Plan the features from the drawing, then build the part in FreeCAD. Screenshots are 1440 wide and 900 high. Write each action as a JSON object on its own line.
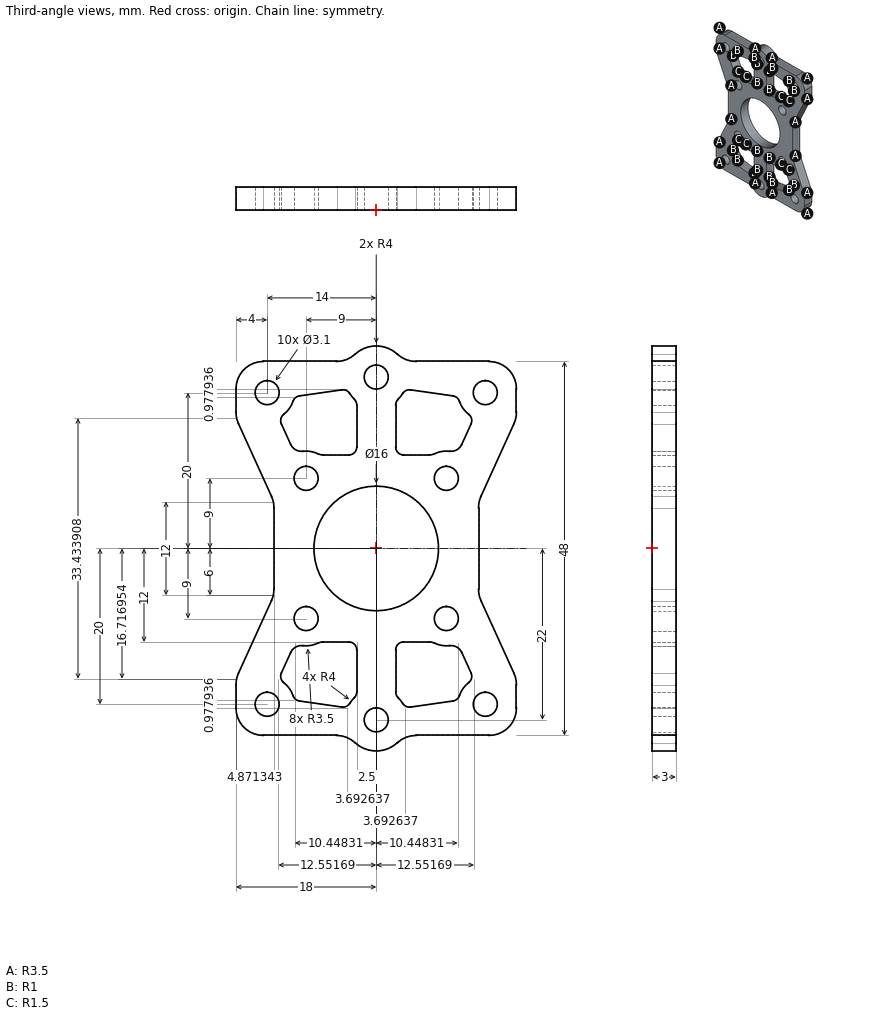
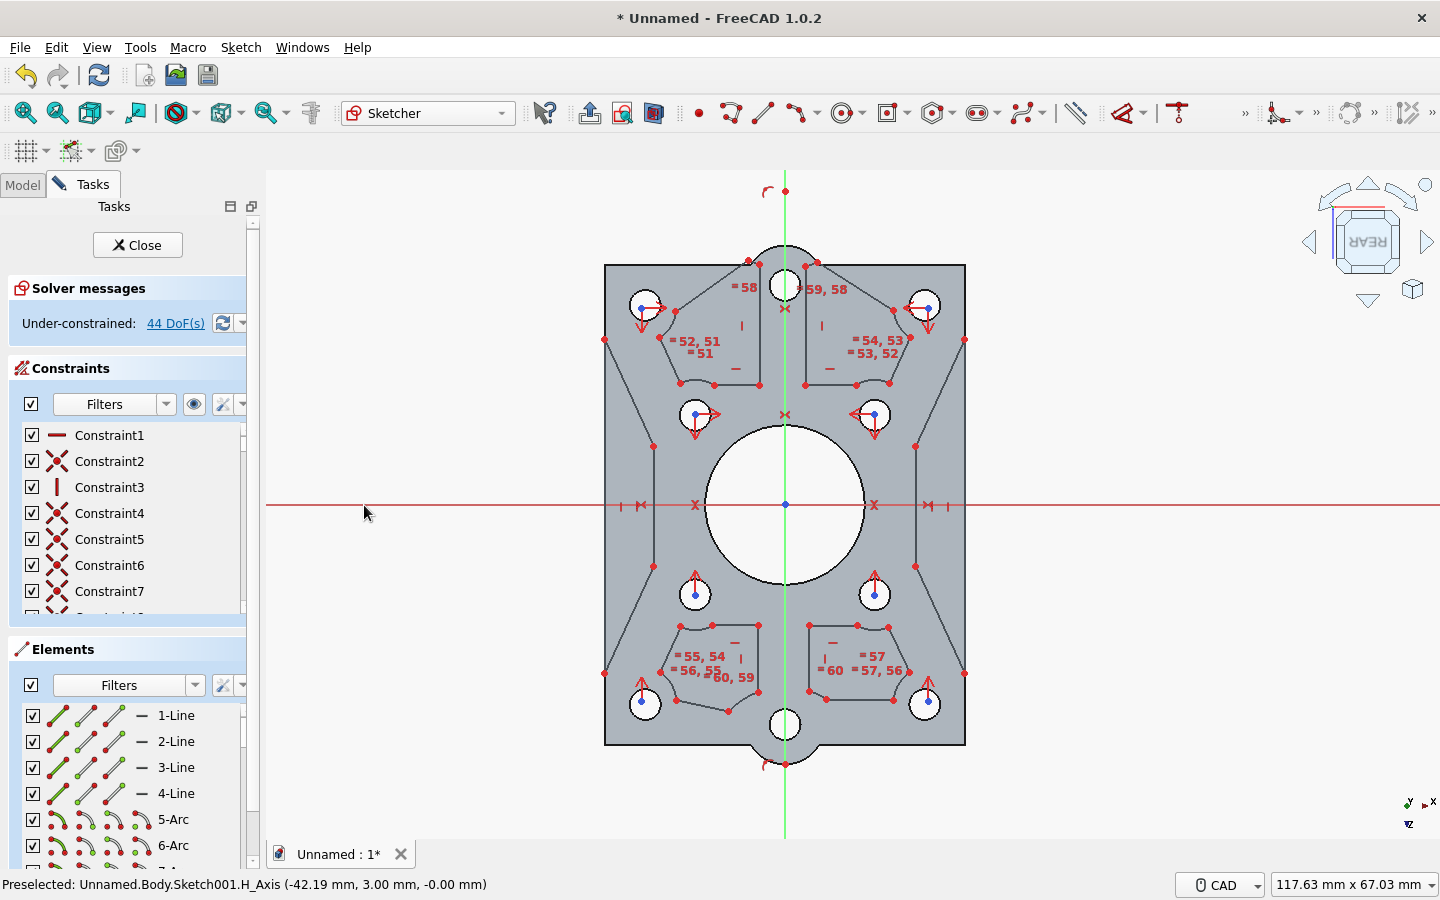
{"action": "left_click", "coordinate": [760, 385]}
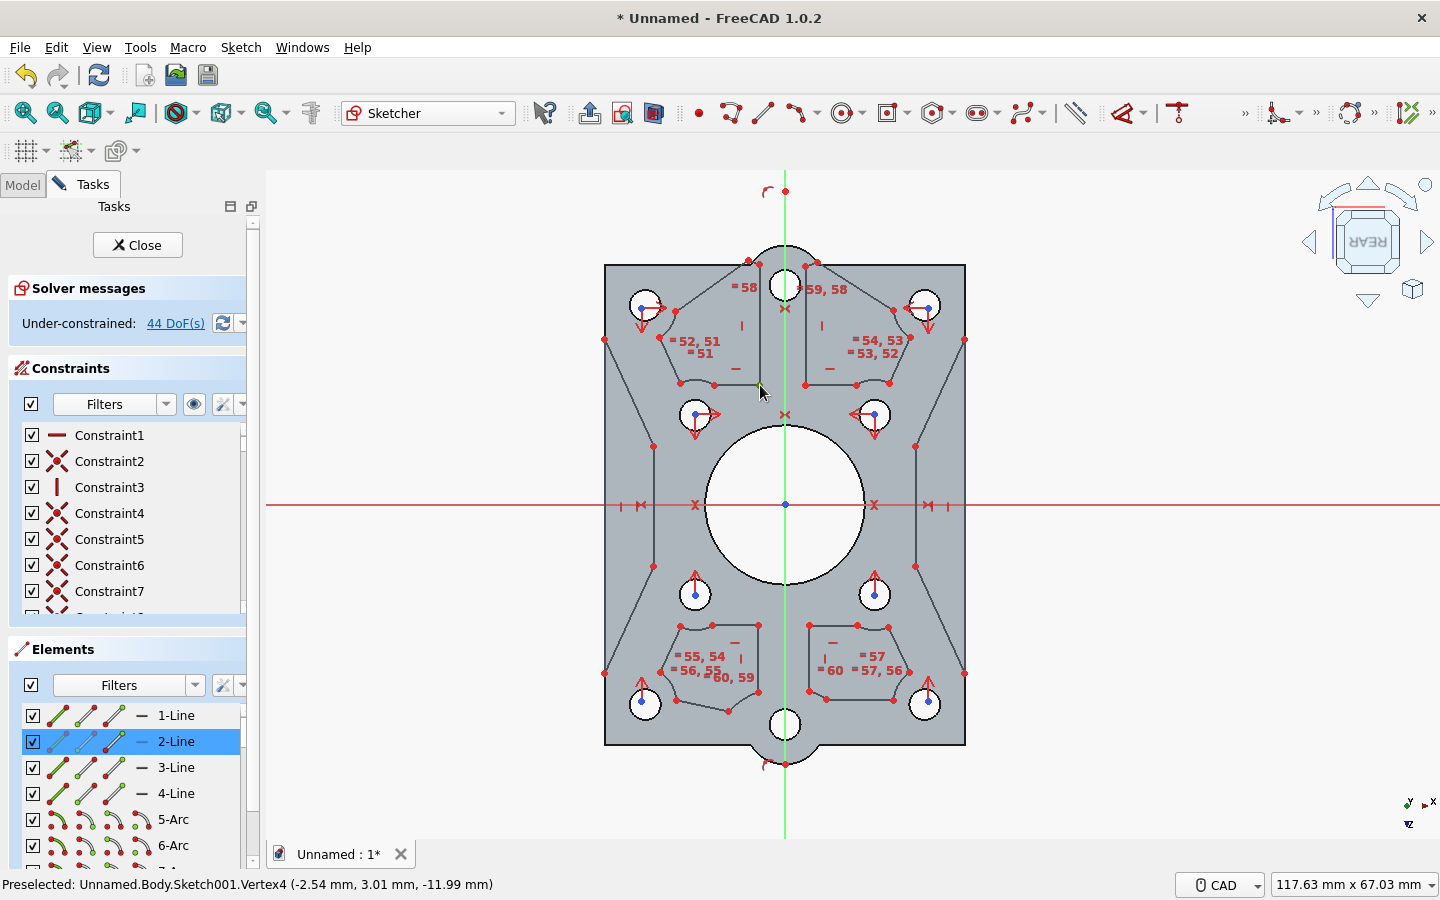
{"action": "left_click", "coordinate": [806, 385]}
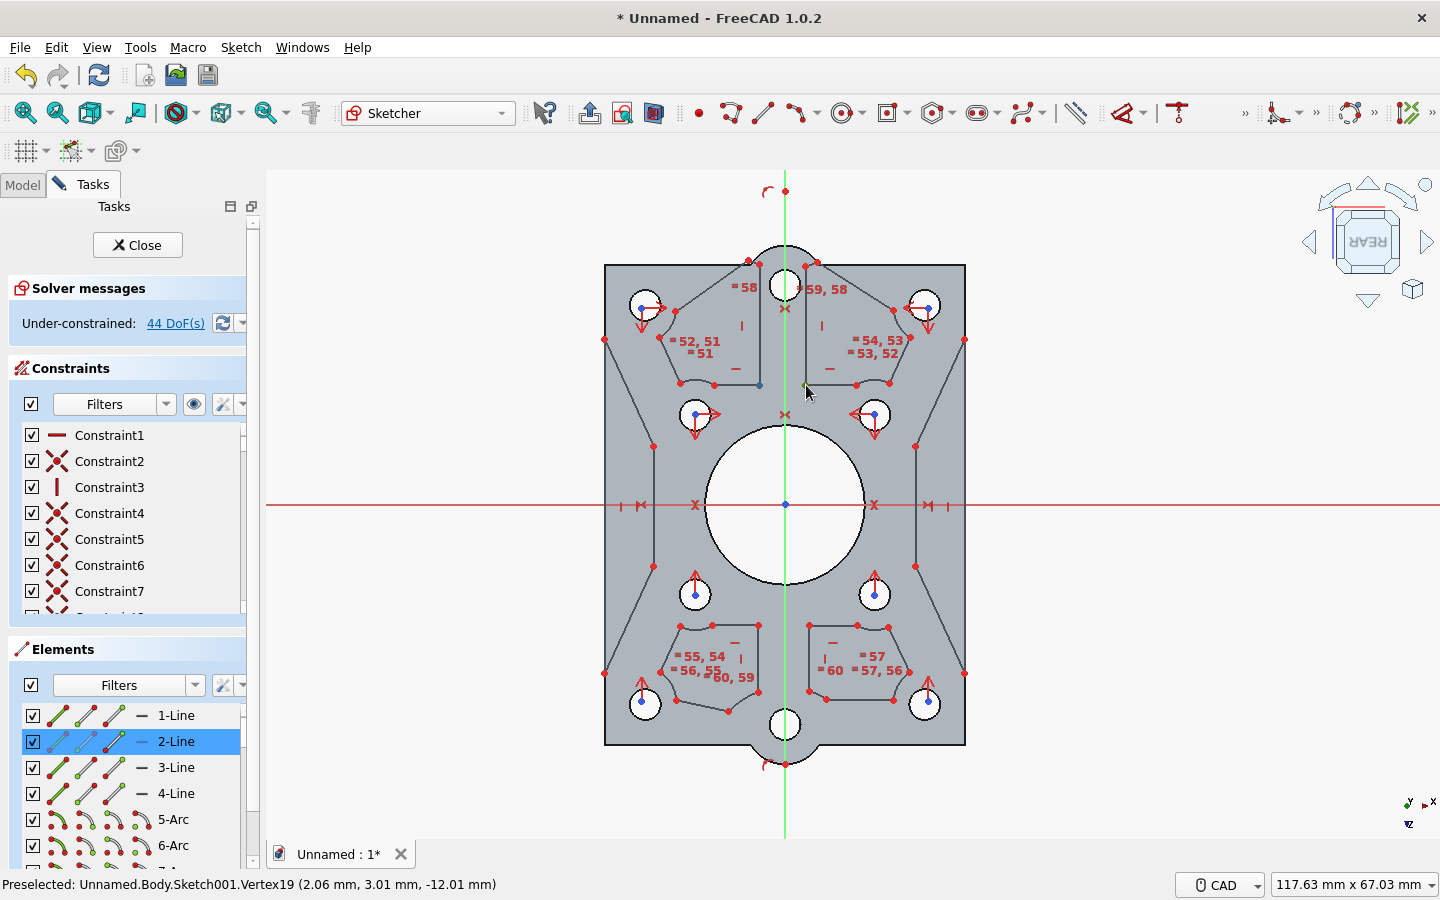
{"action": "left_click", "coordinate": [785, 723]}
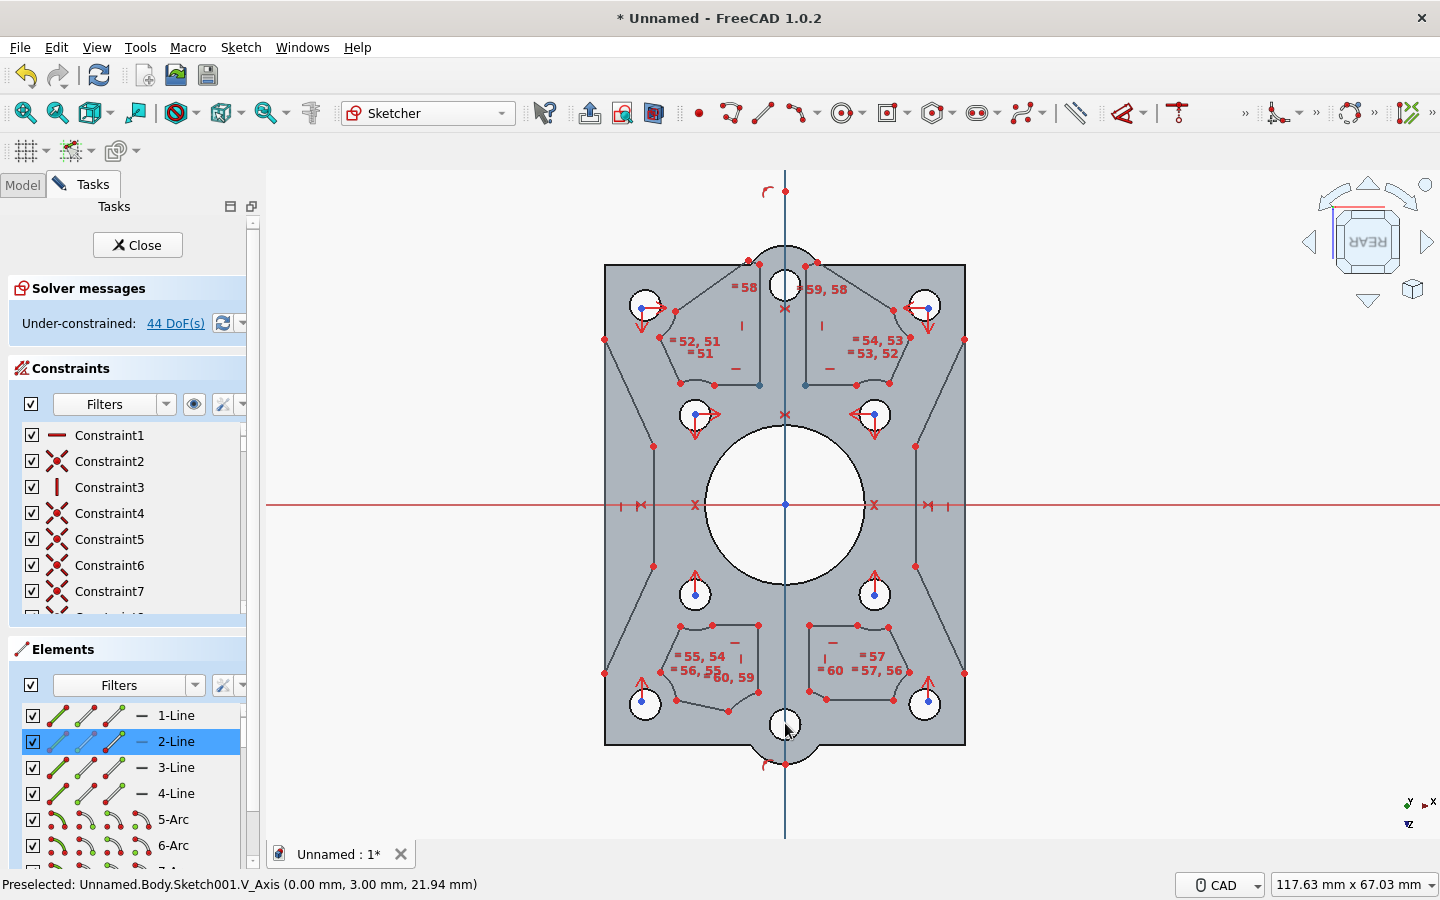
{"action": "key", "text": "s"}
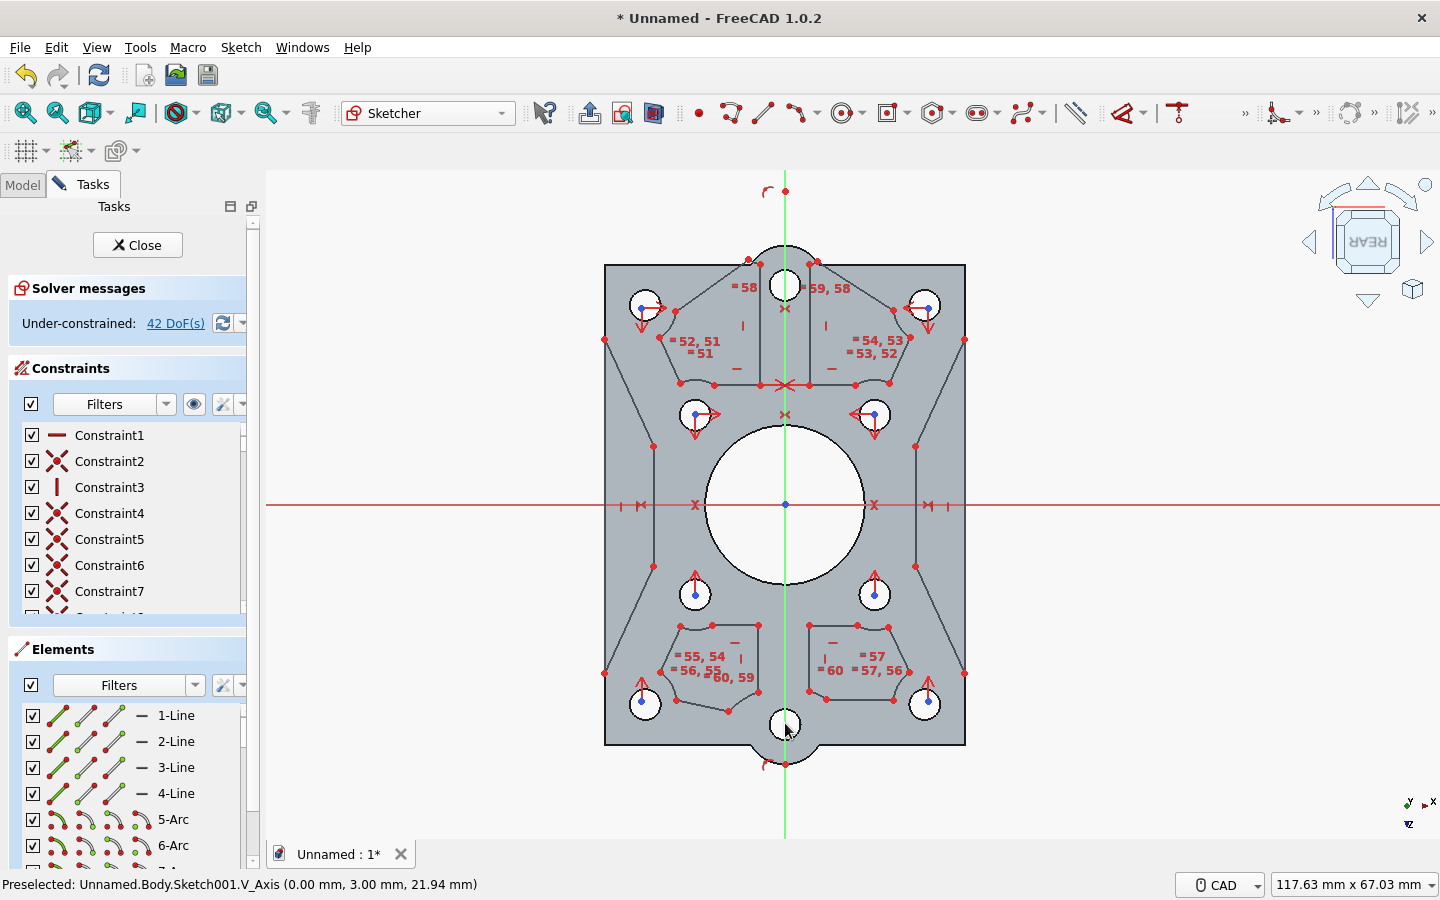
{"action": "left_click", "coordinate": [654, 446]}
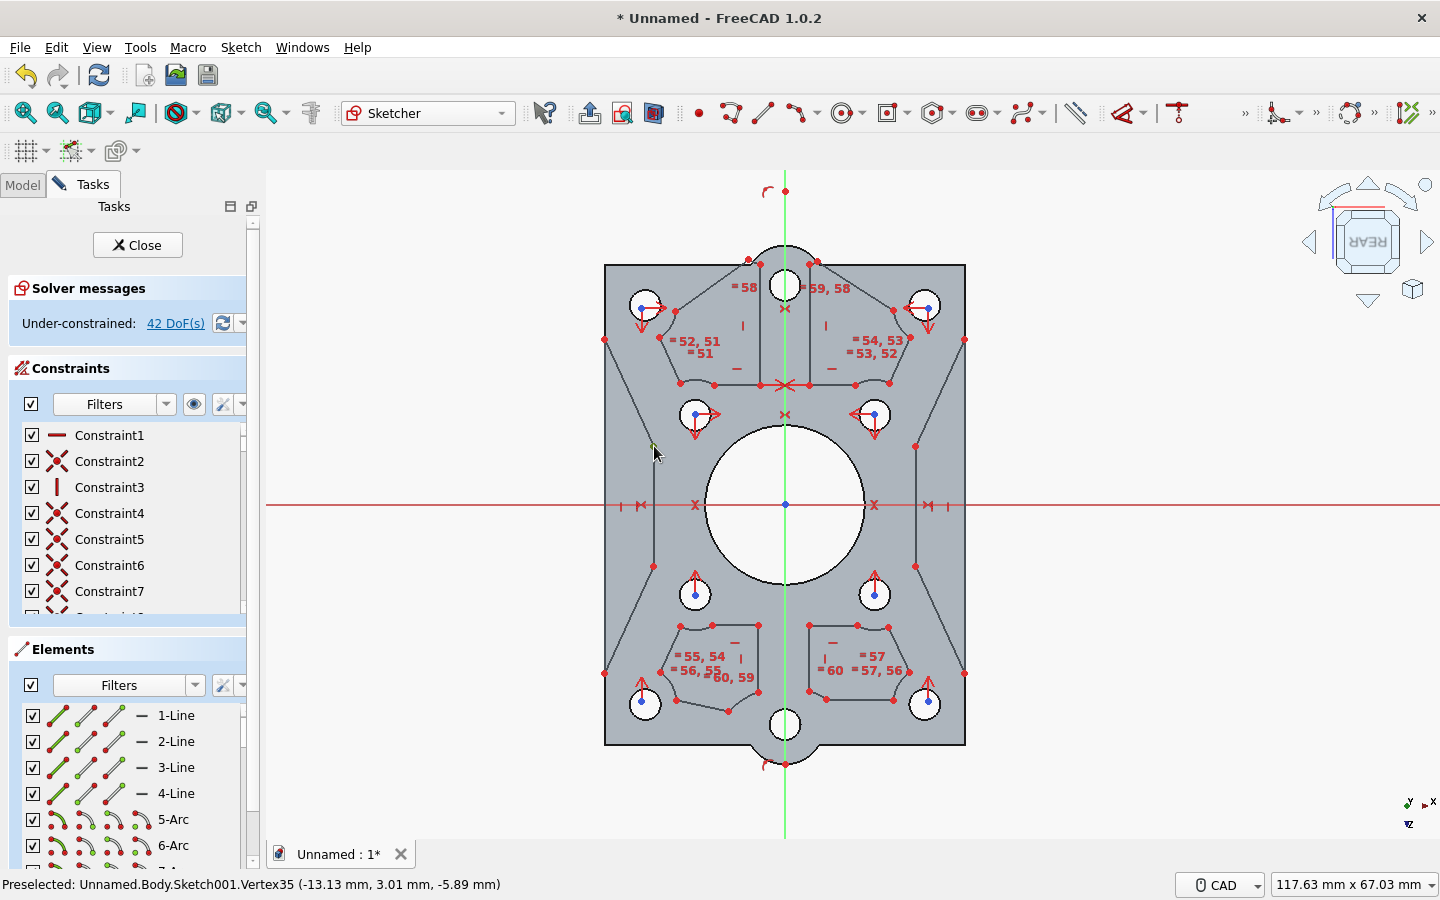
{"action": "left_click", "coordinate": [916, 446]}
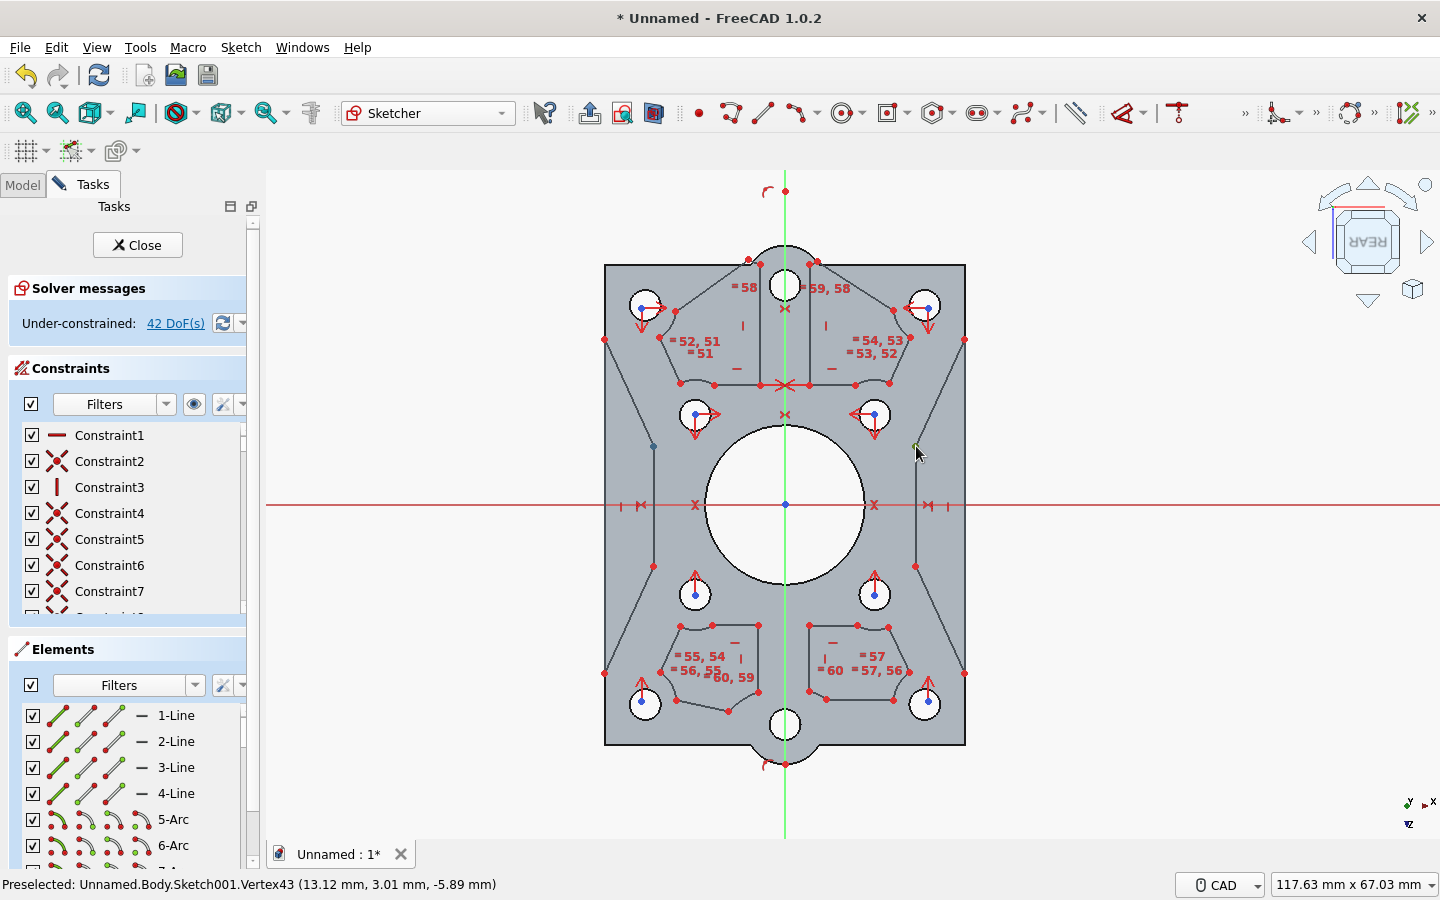
{"action": "left_click", "coordinate": [785, 723]}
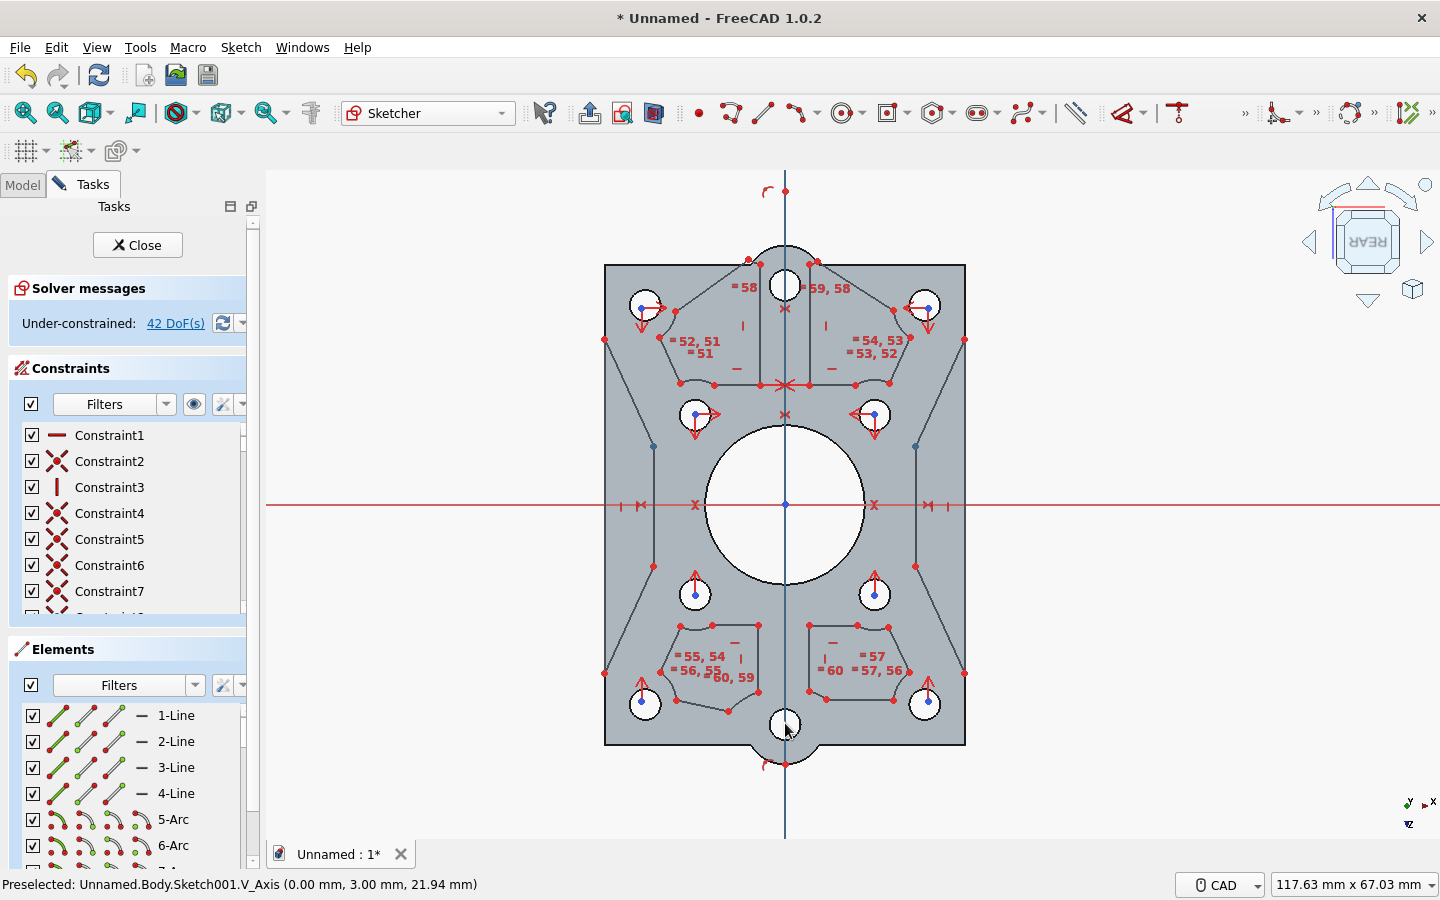
{"action": "key", "text": "s"}